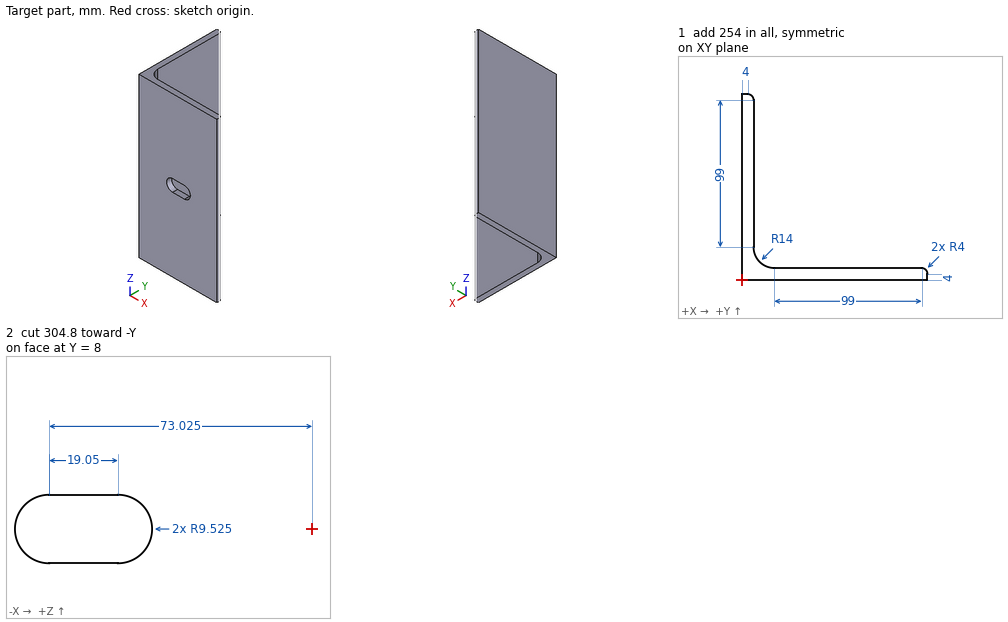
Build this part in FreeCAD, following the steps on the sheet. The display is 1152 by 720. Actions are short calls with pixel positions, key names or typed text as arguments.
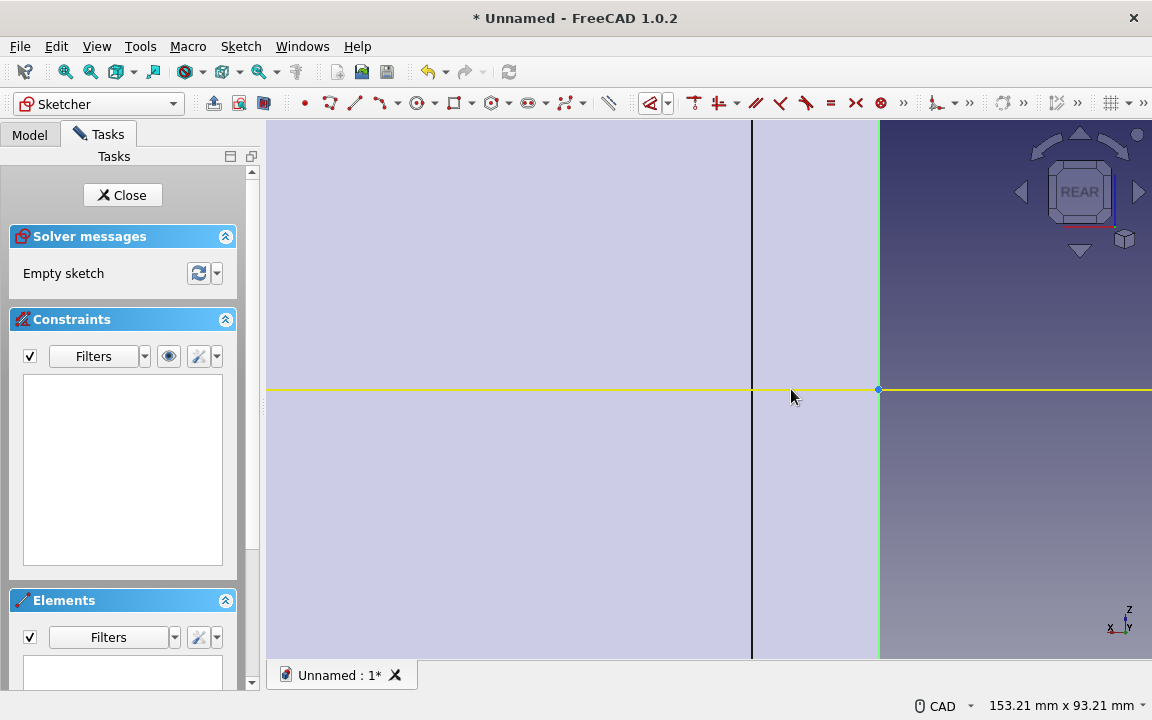
key(g)
key(s)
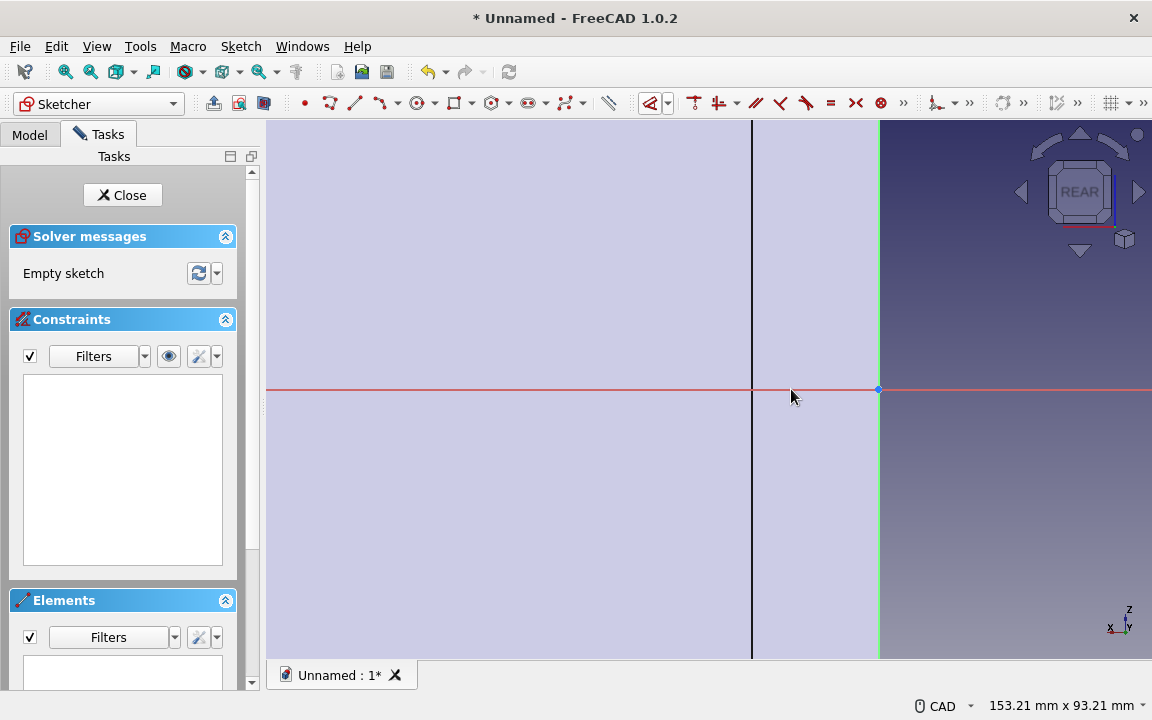
click(457, 389)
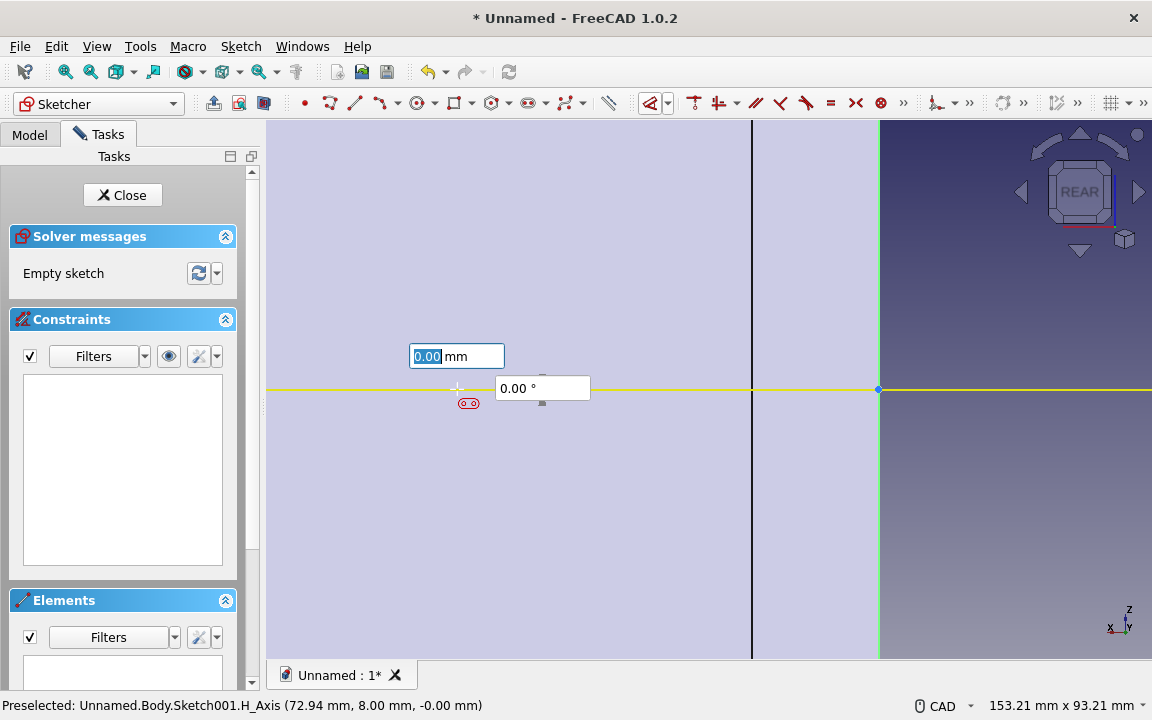
click(567, 380)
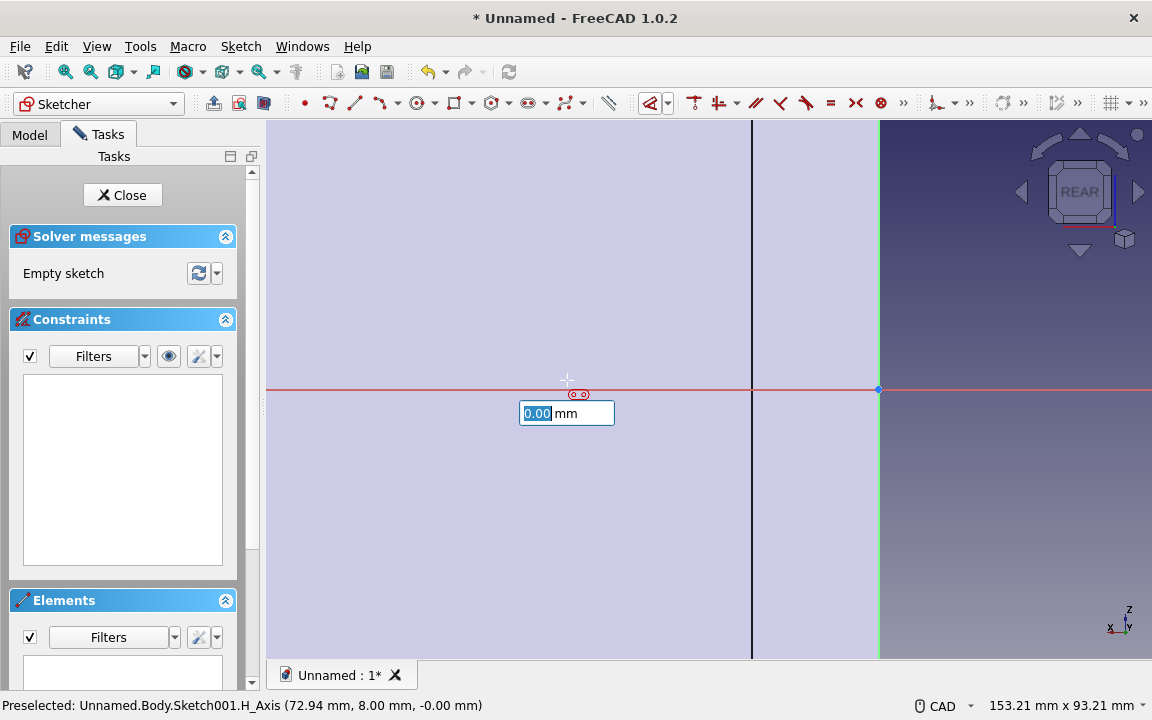
click(512, 445)
key(Escape)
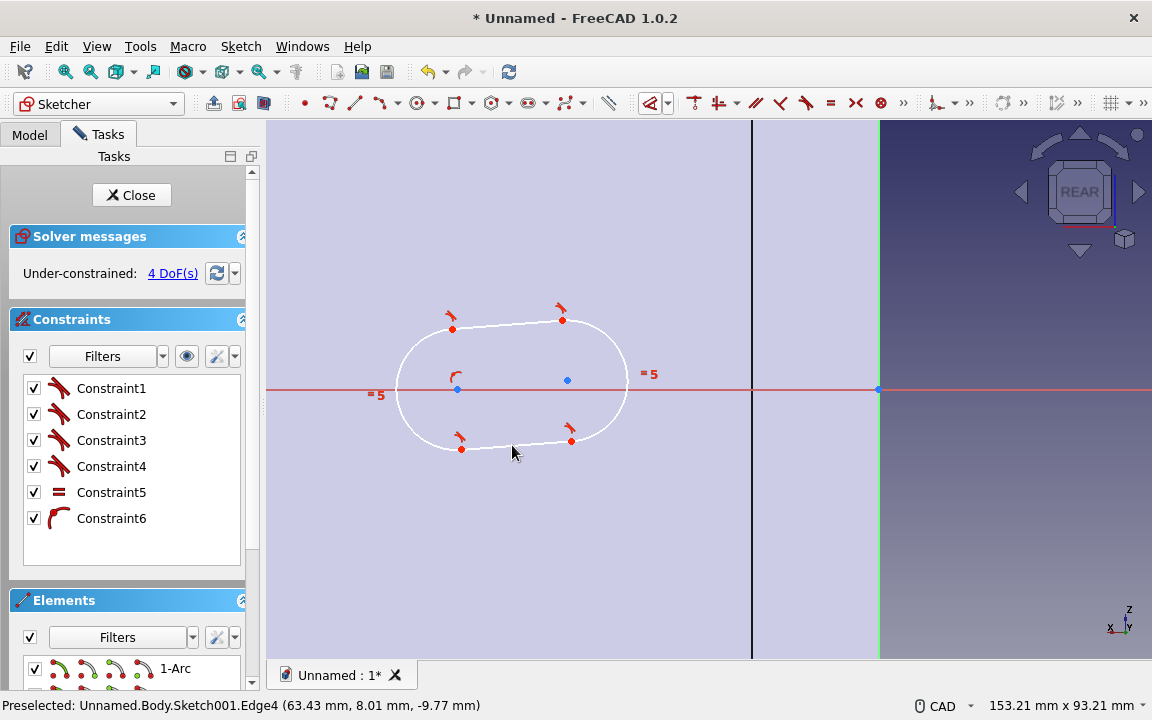
click(485, 327)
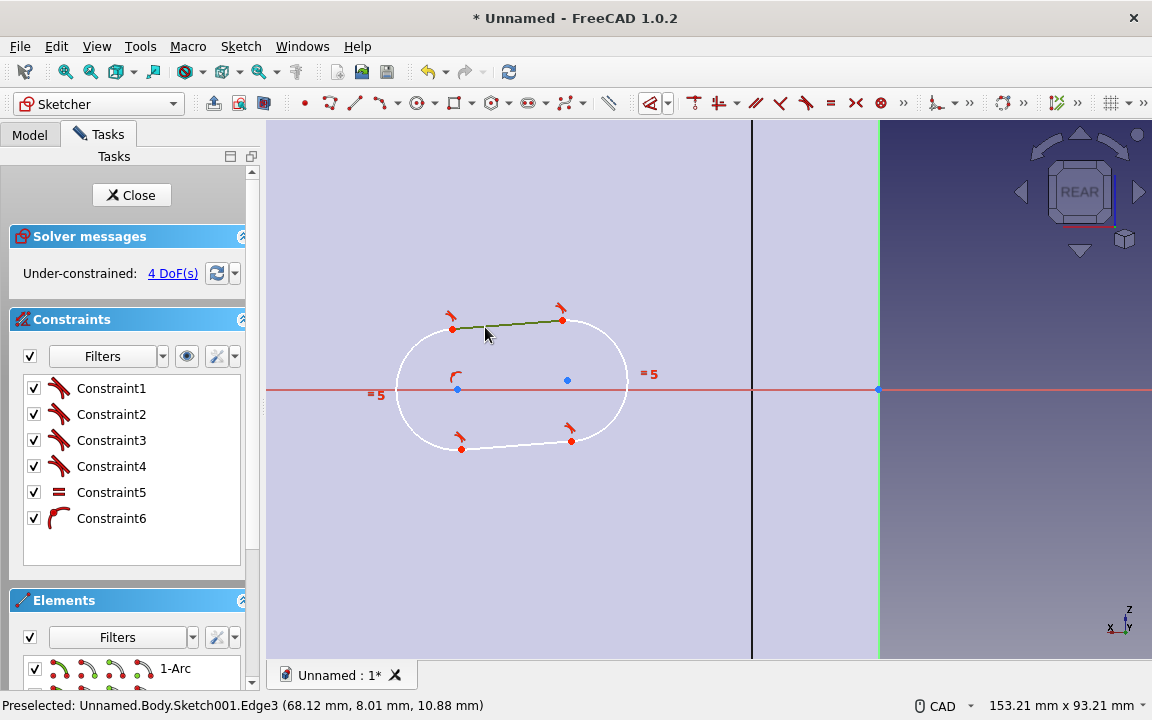
click(736, 104)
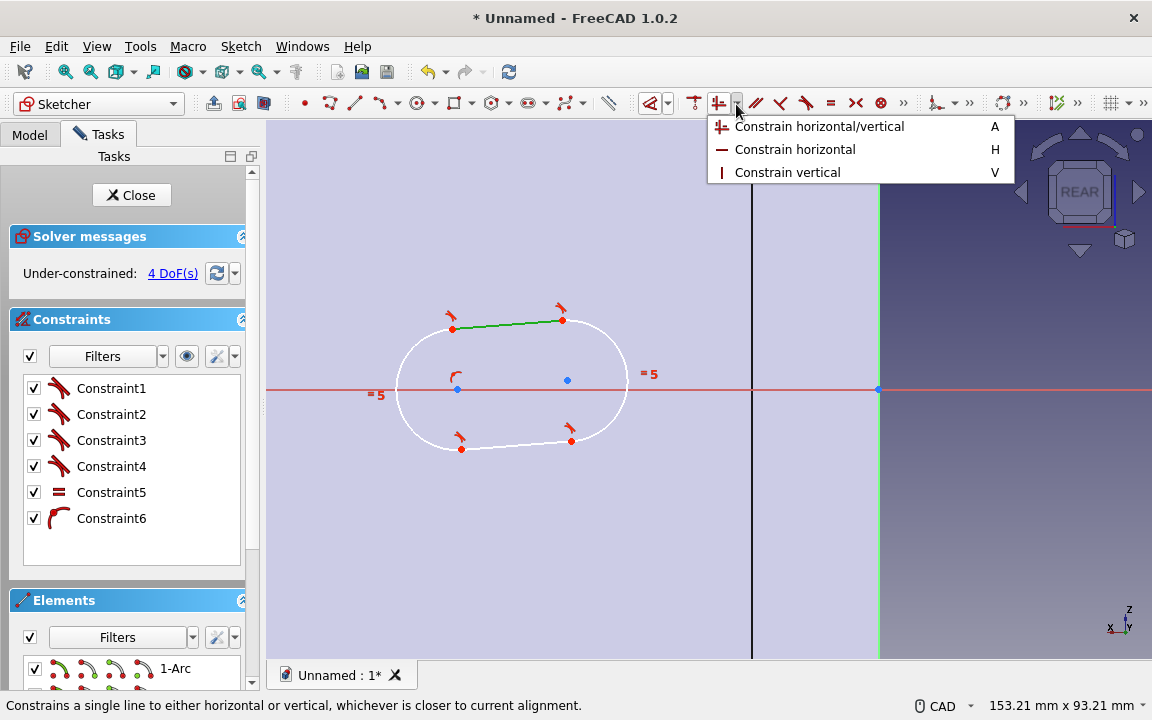
click(861, 150)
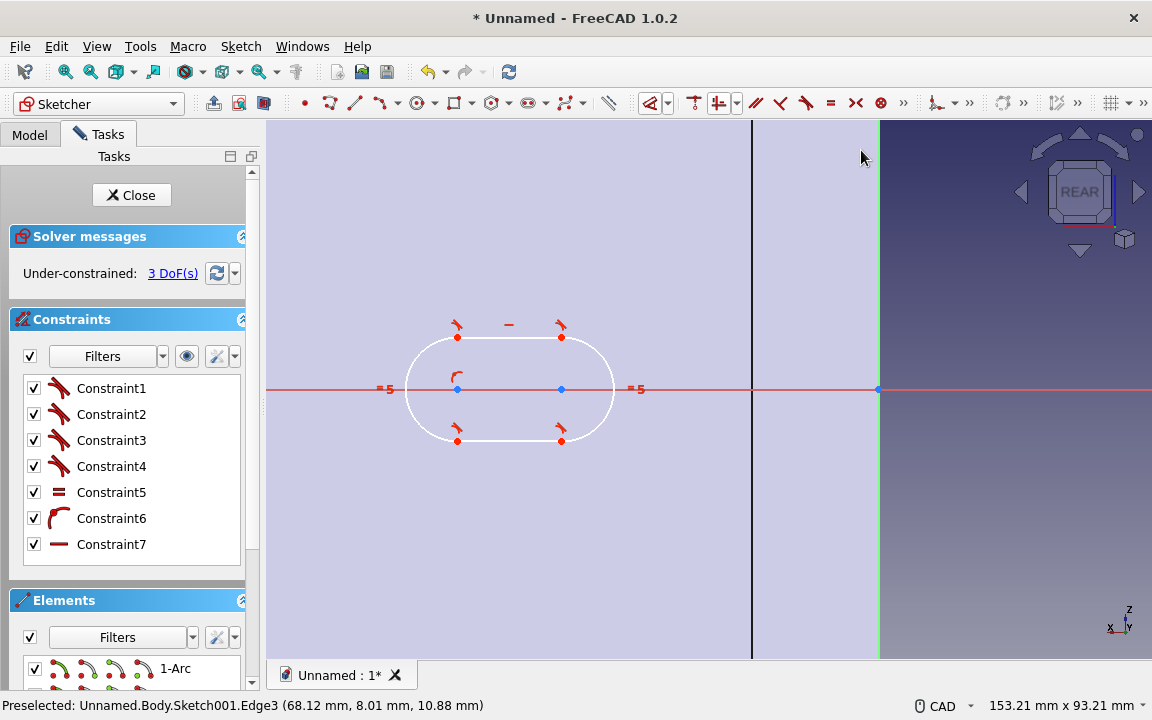
click(416, 359)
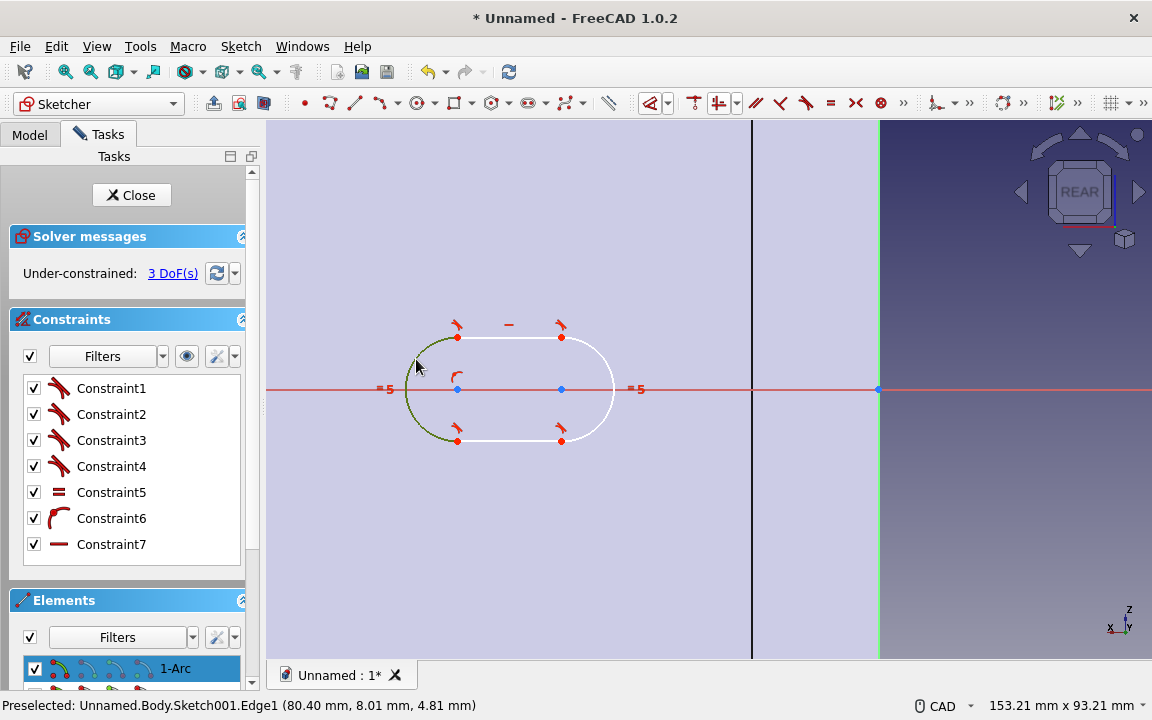
key(k)
key(r)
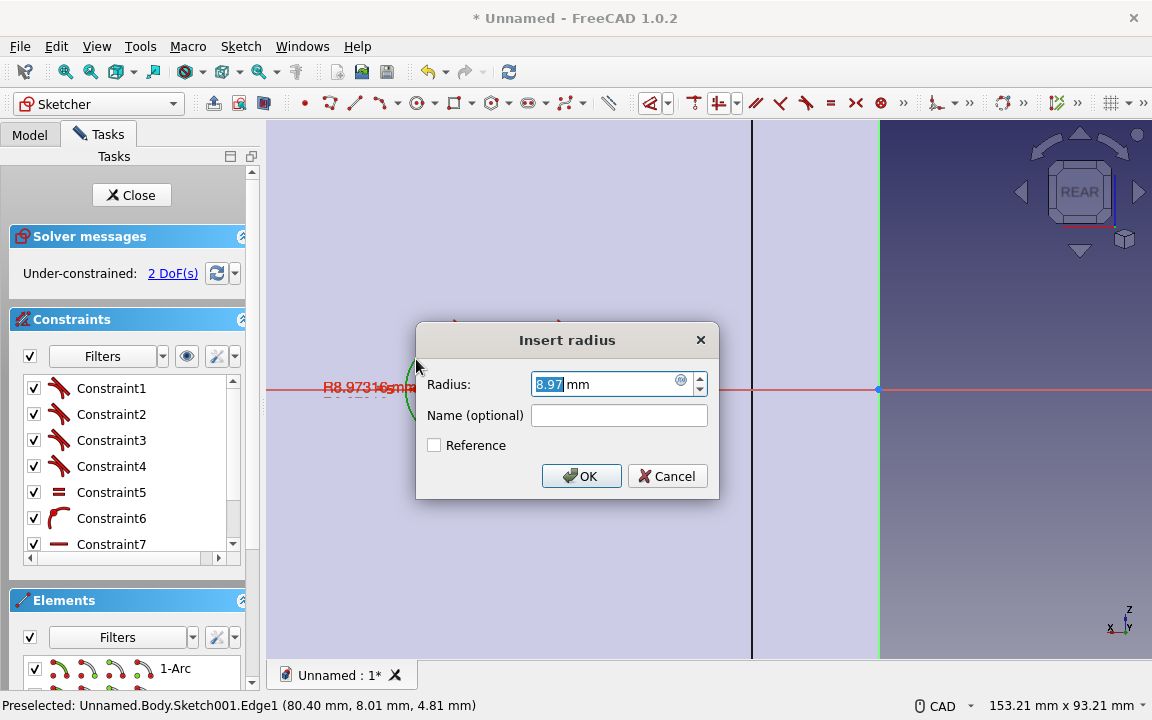
text(9.525)
key(Return)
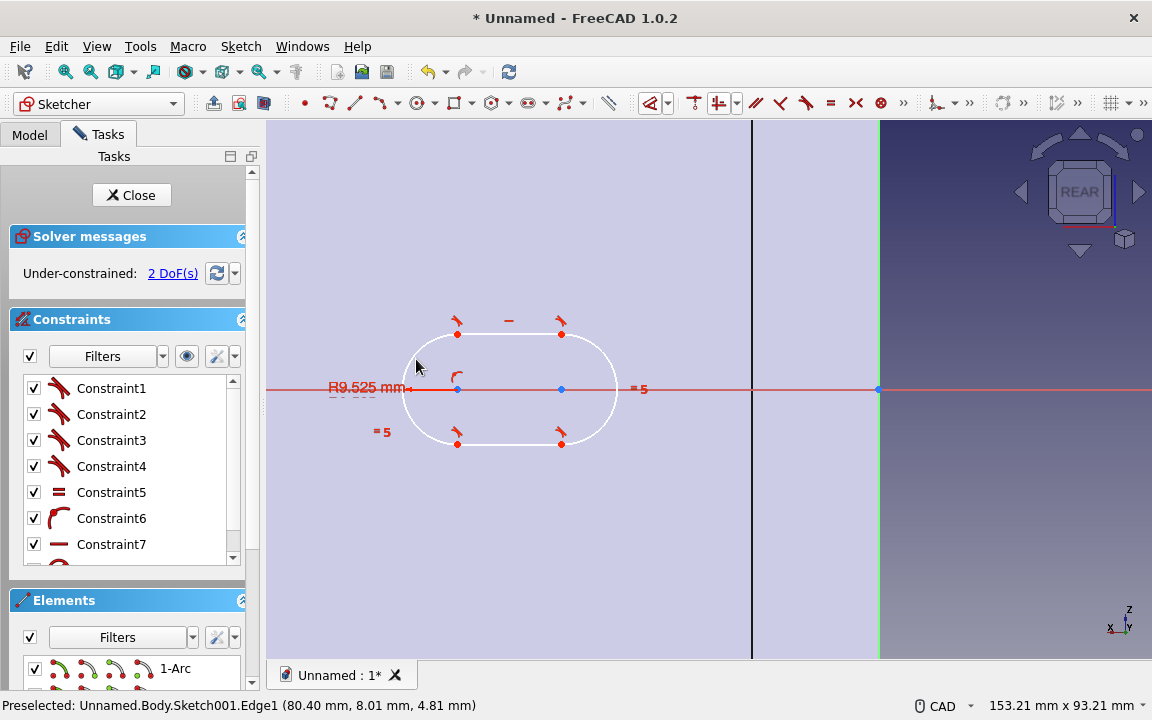
click(489, 334)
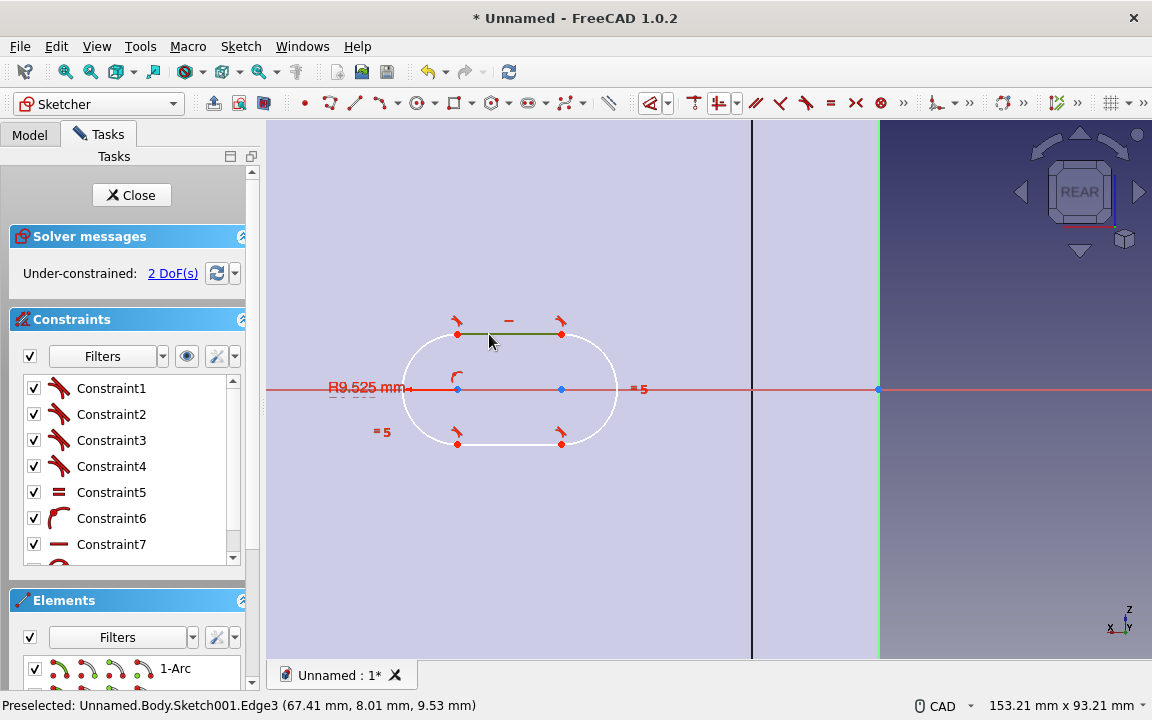
click(668, 104)